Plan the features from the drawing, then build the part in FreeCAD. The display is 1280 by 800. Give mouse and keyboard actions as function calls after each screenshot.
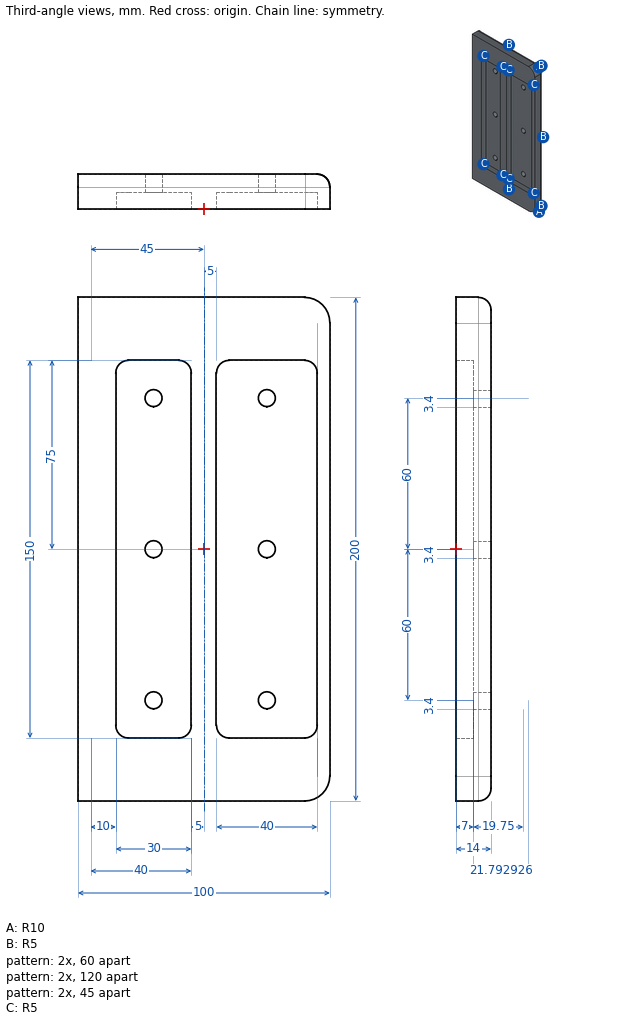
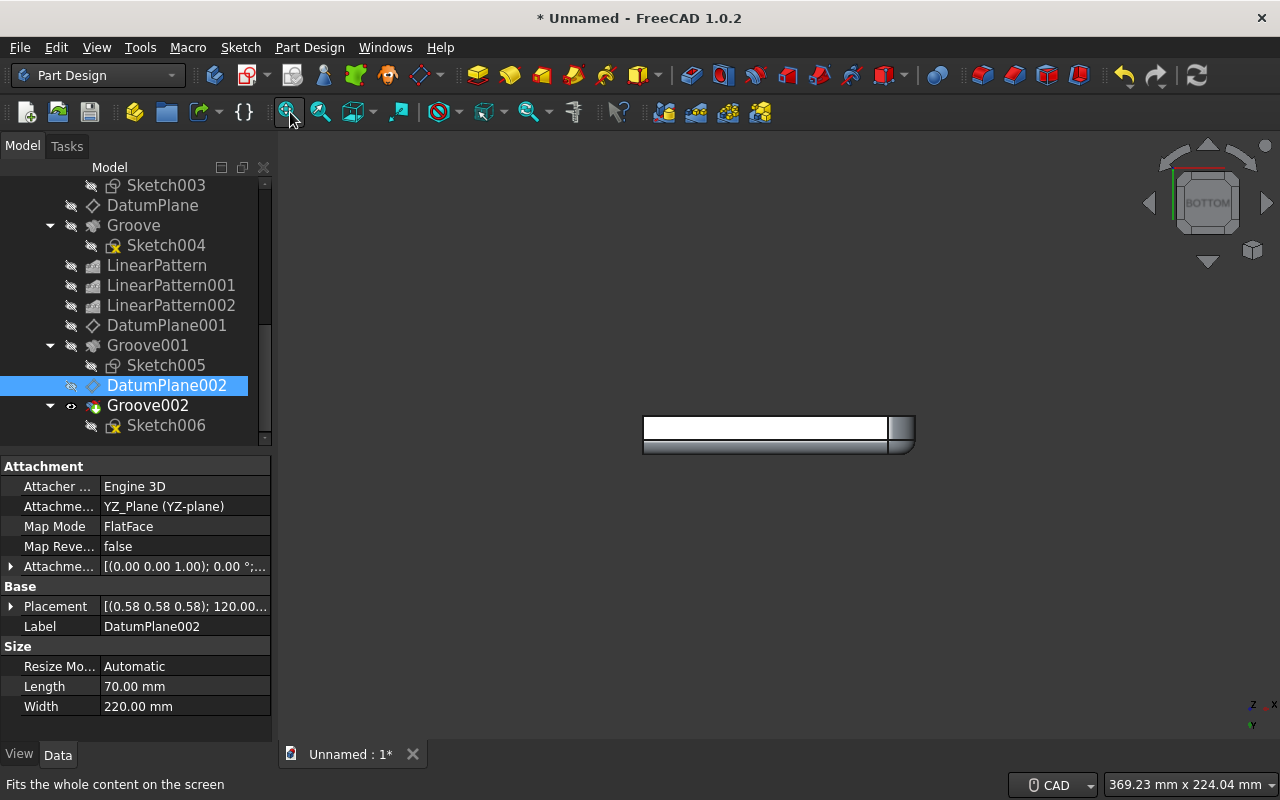
key(4)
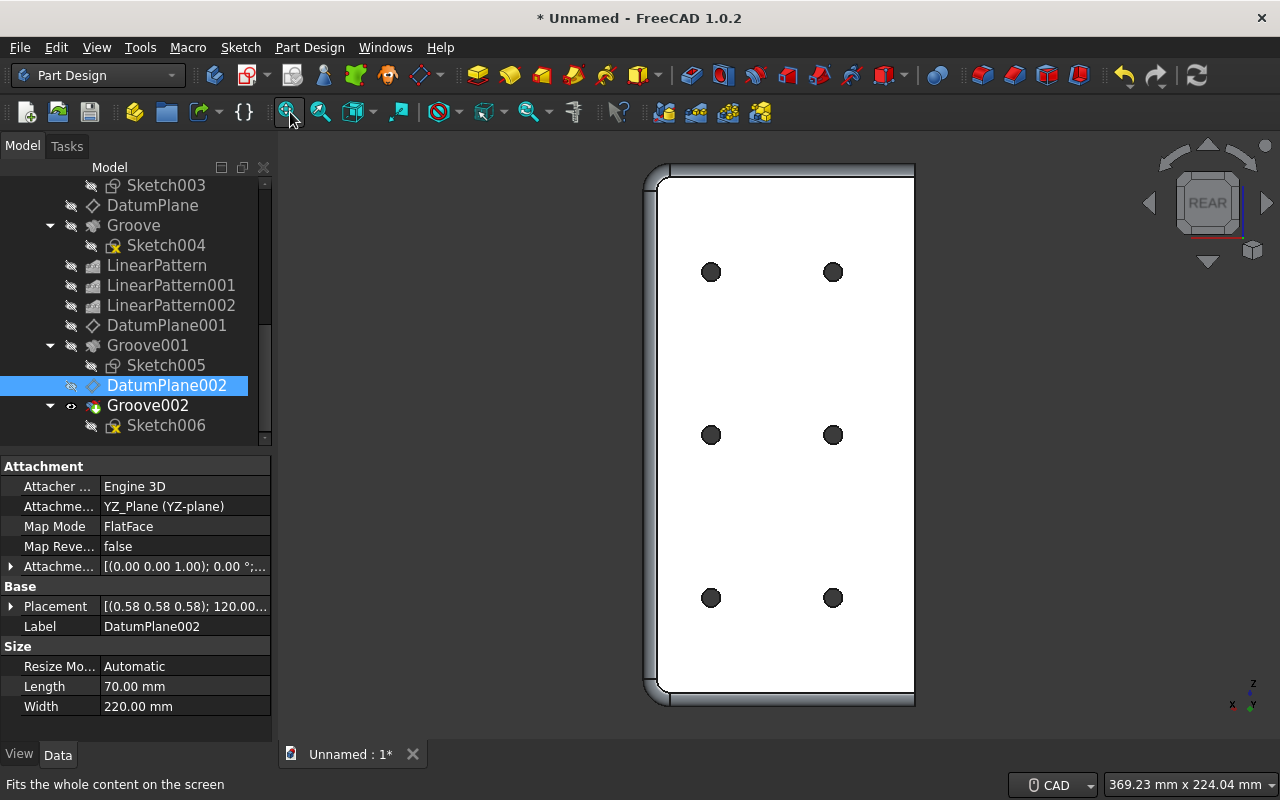
scroll(657, 230, up, 4)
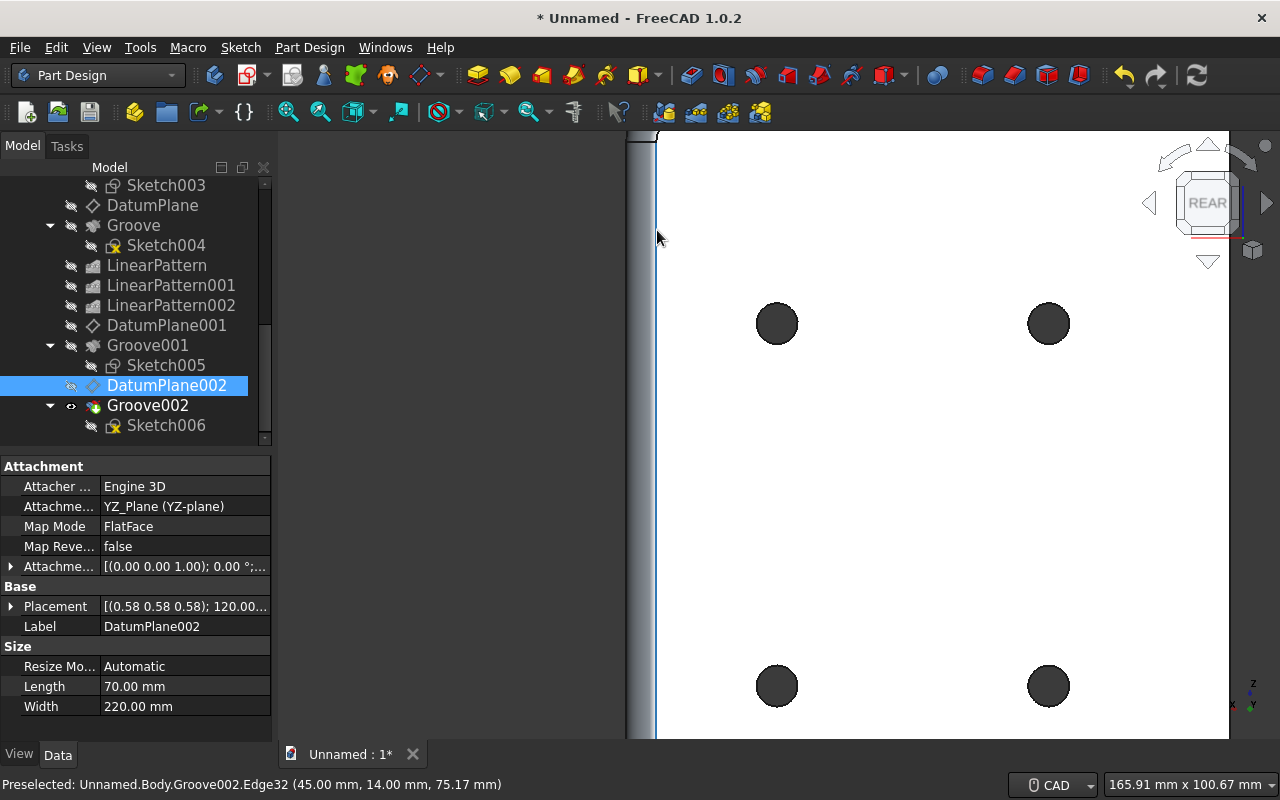
click(290, 112)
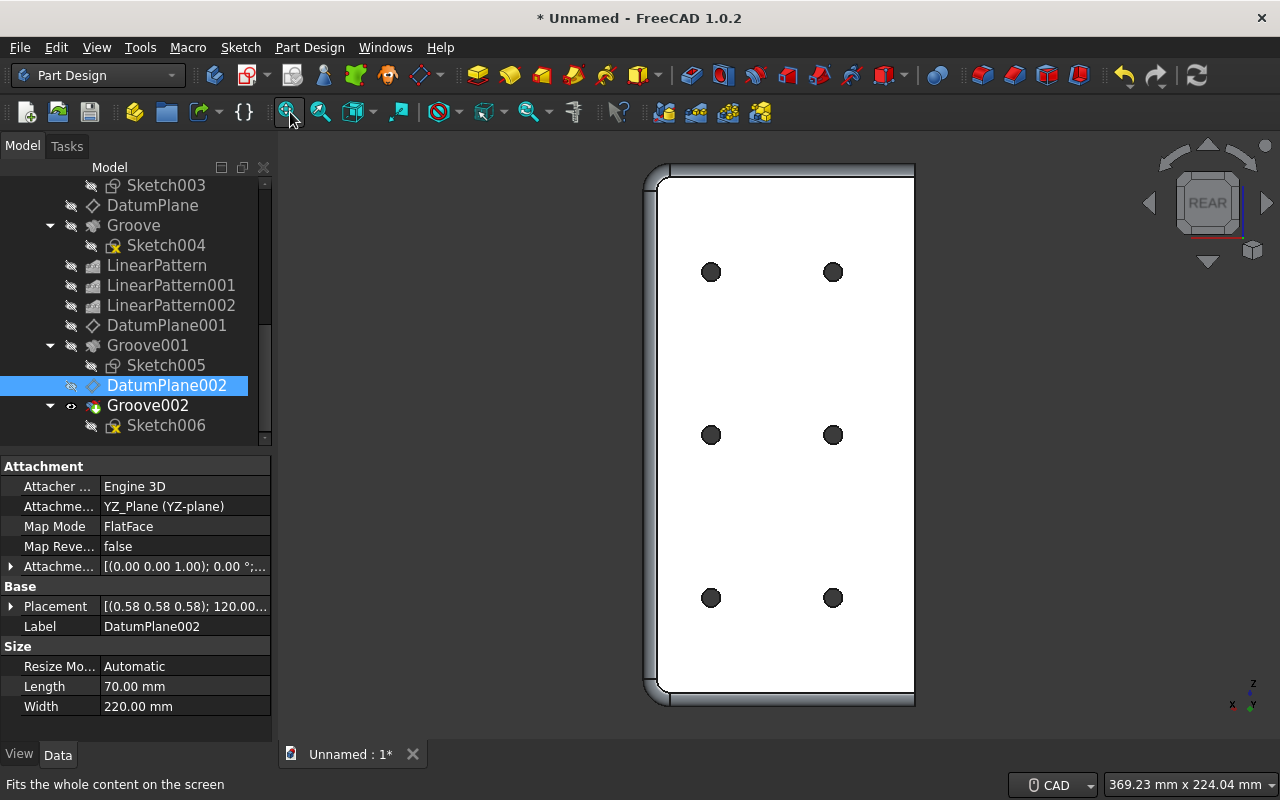
key(6)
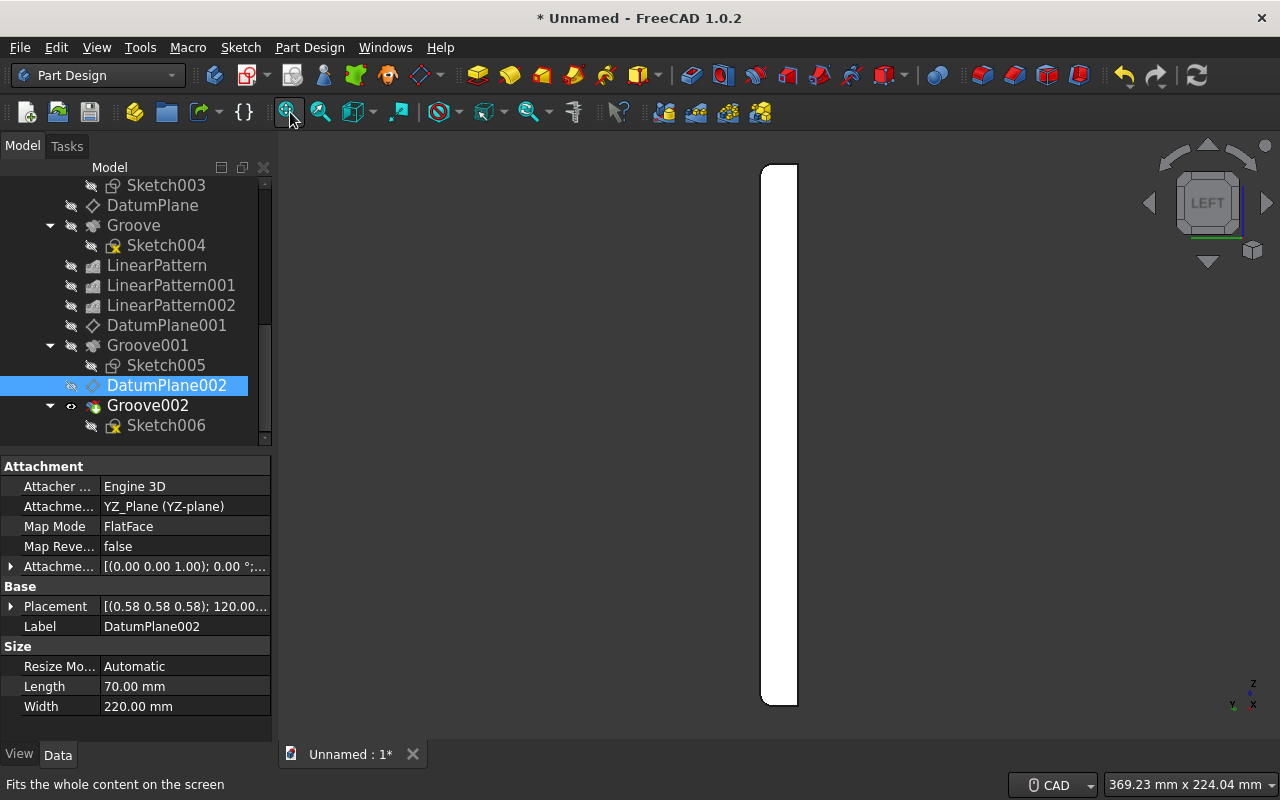
scroll(788, 230, up, 4)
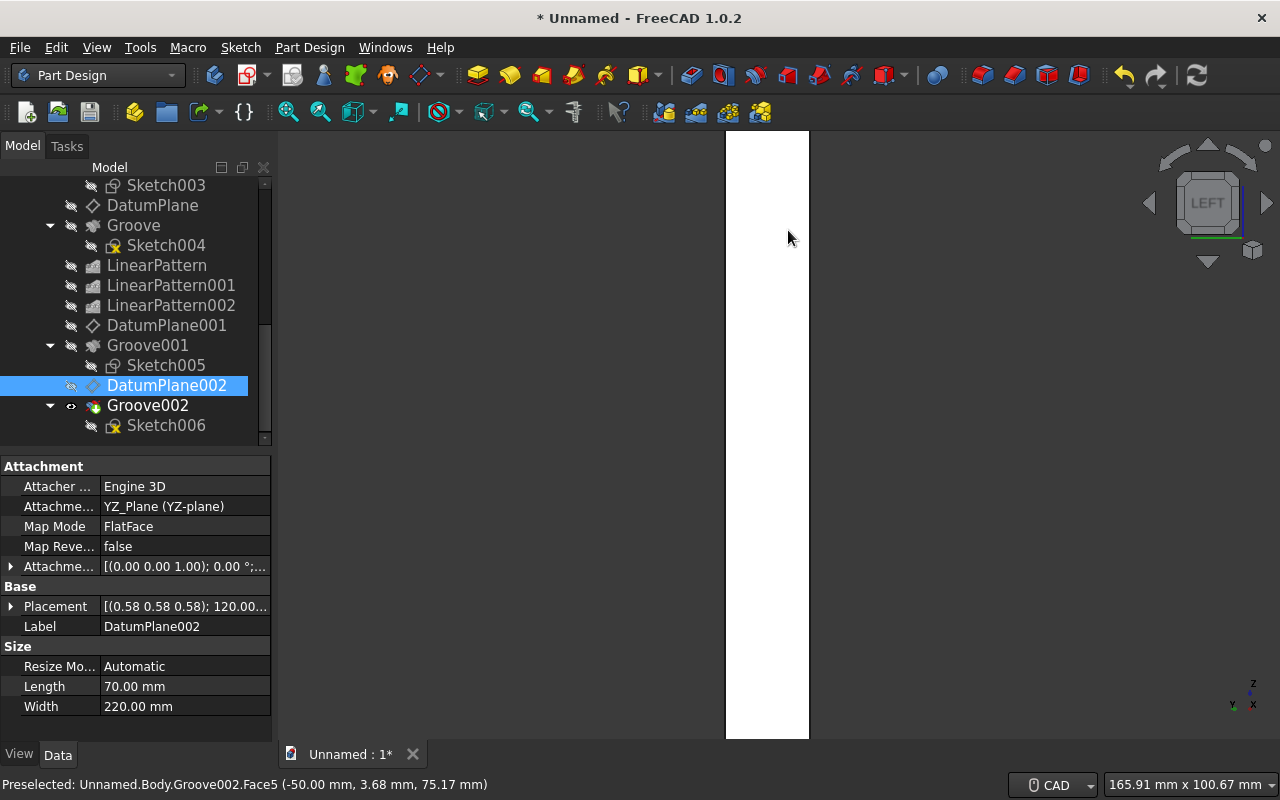
click(290, 112)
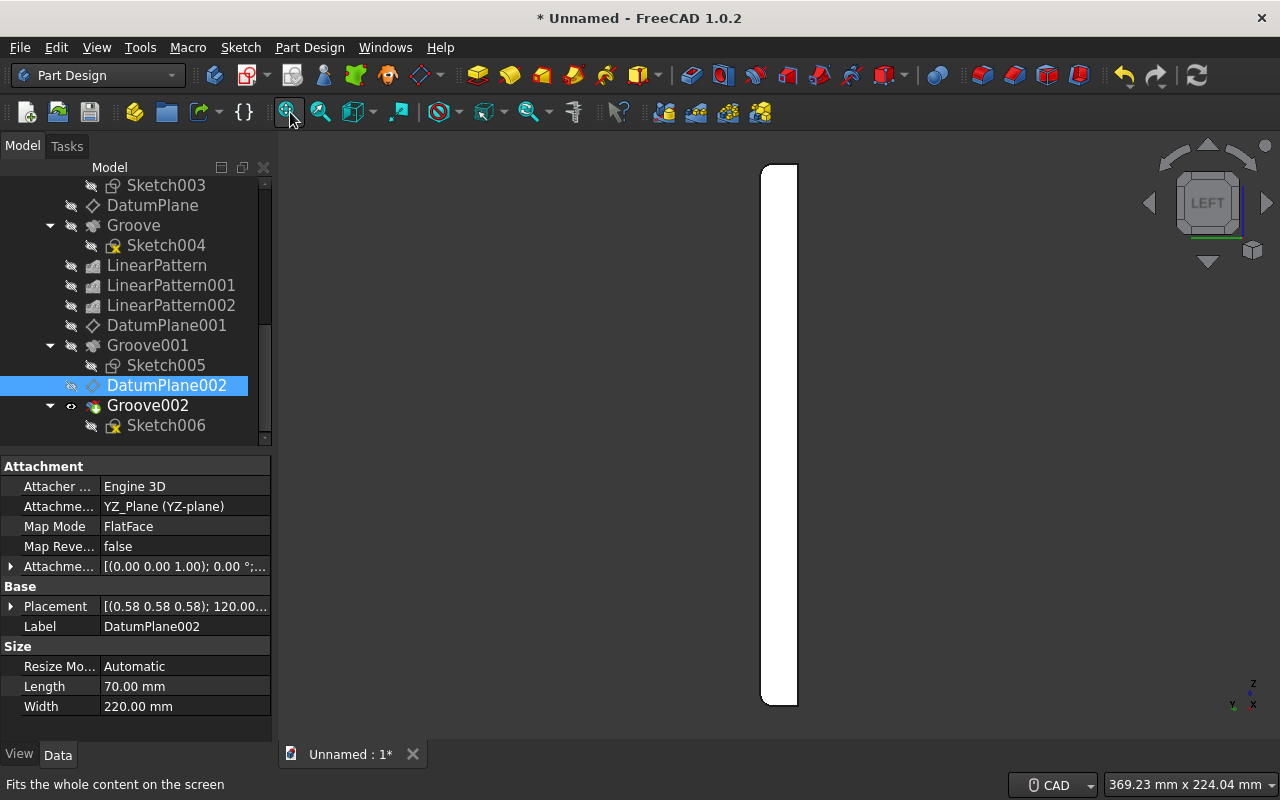
key(v)
key(3)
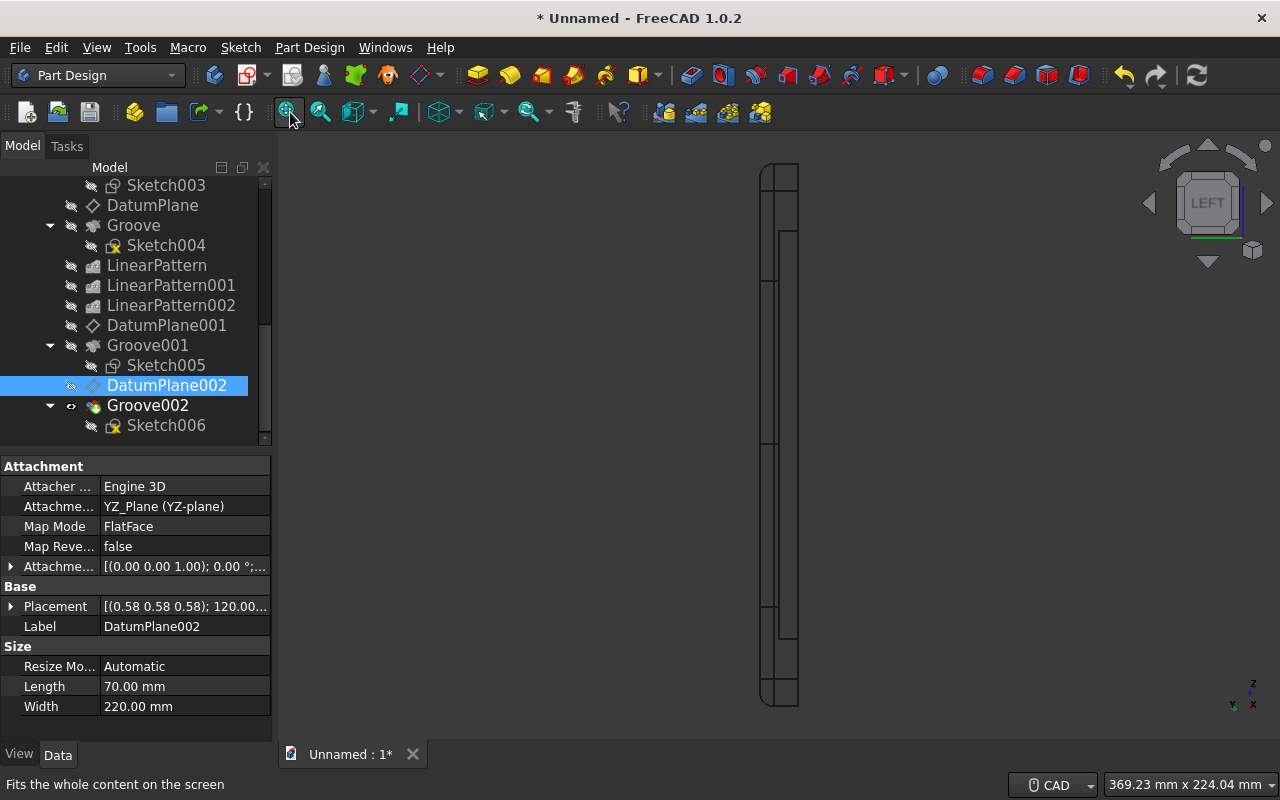
key(0)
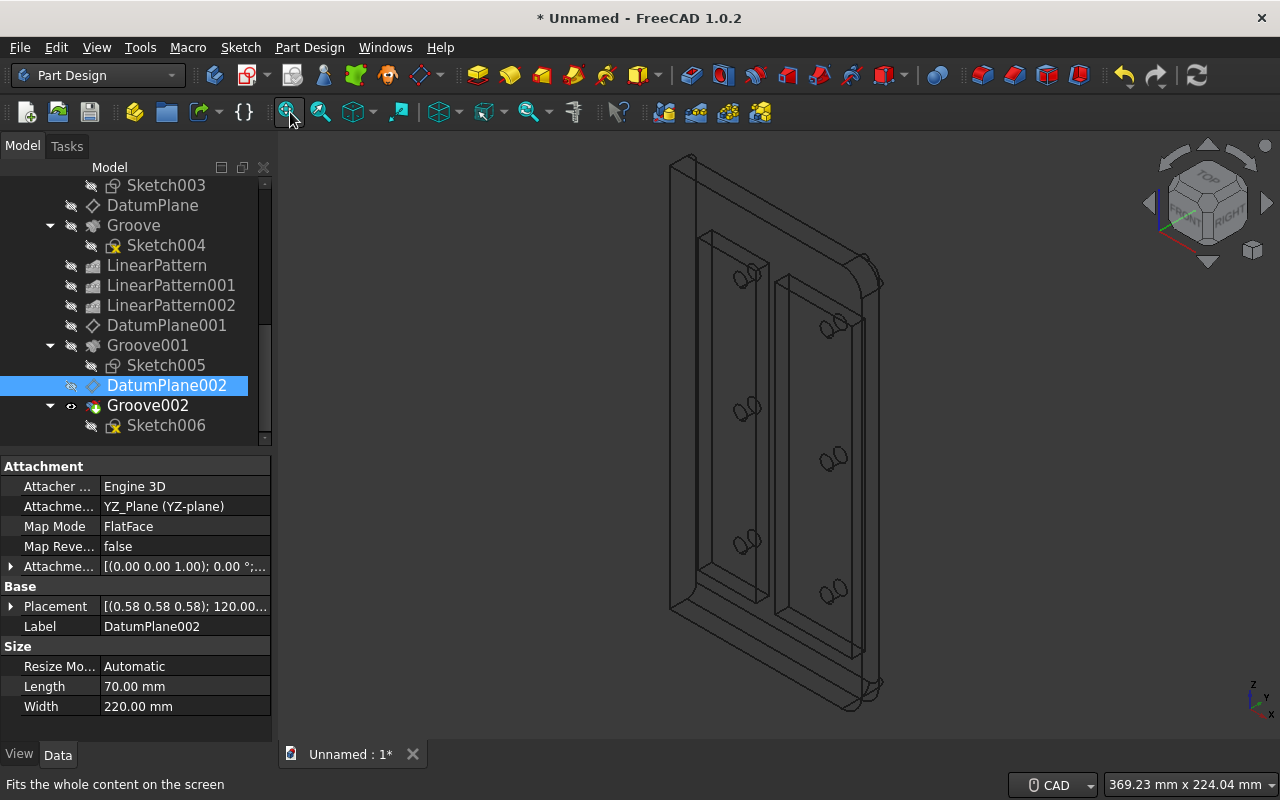
click(782, 610)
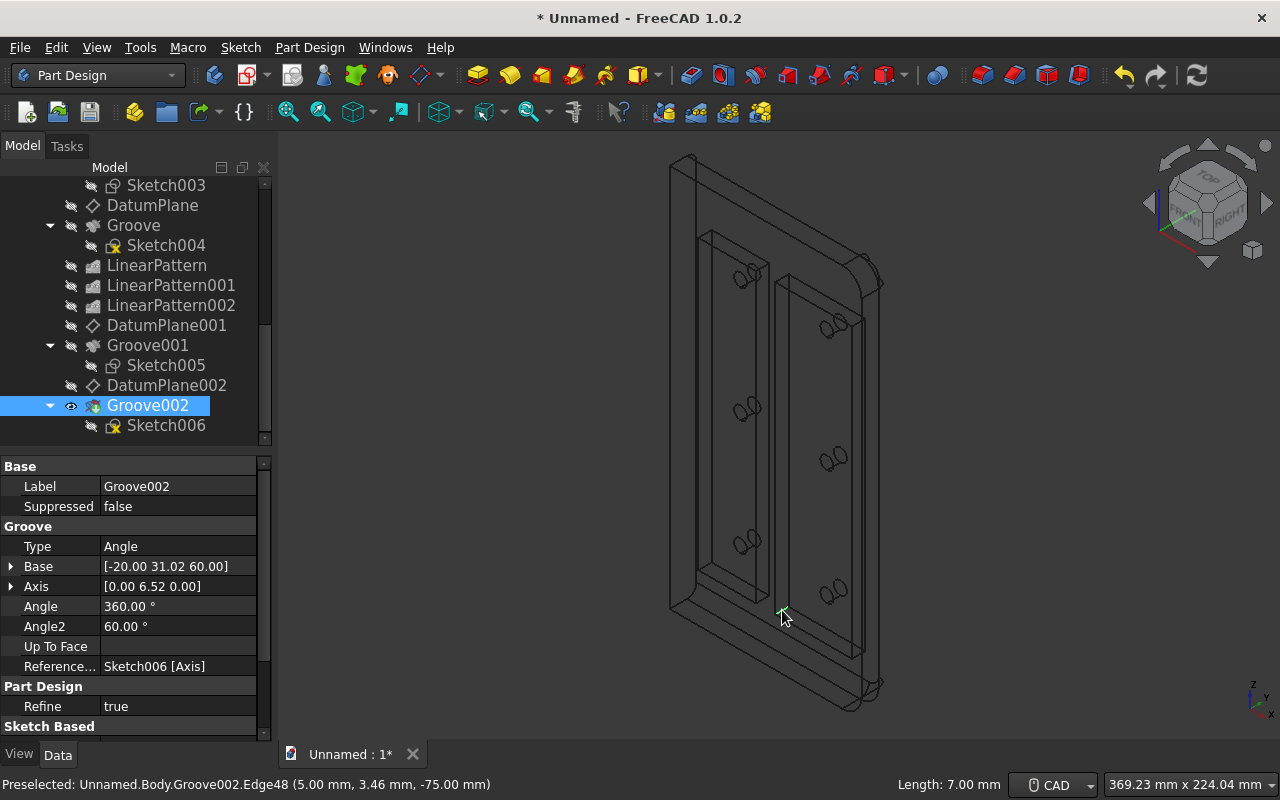
click(782, 277, ctrl)